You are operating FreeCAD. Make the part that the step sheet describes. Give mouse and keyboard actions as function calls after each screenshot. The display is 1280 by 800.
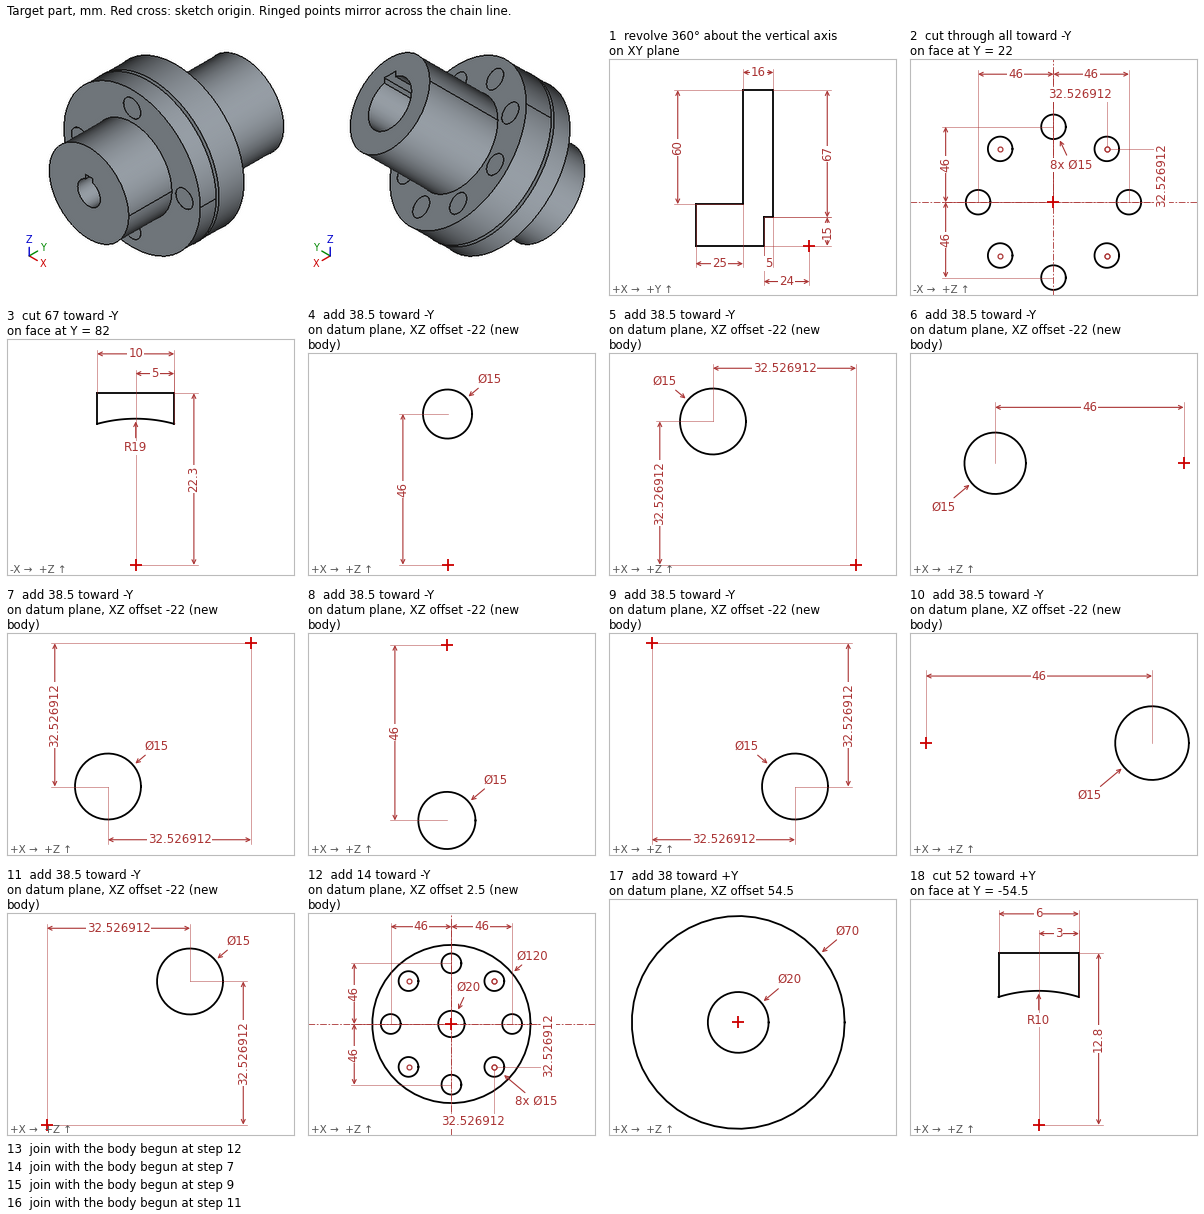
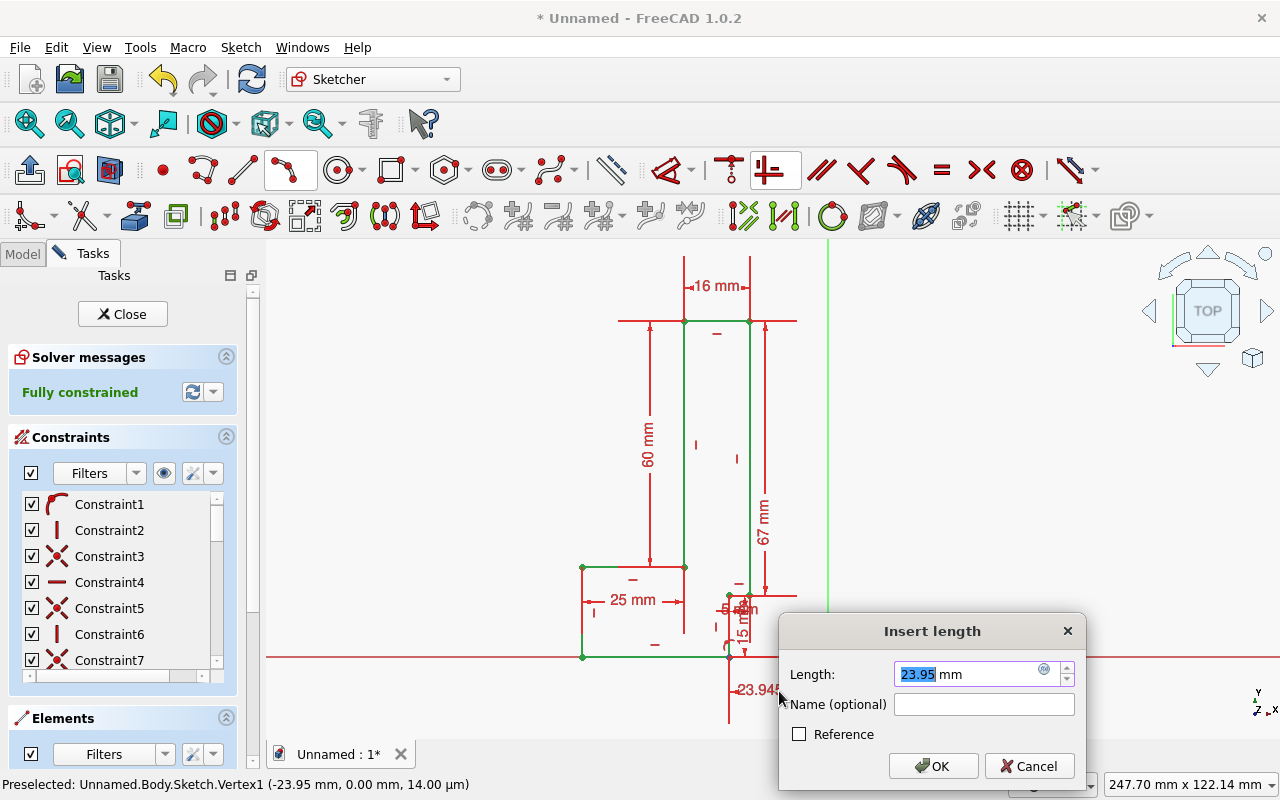
text(24)
key(Return)
key(Escape)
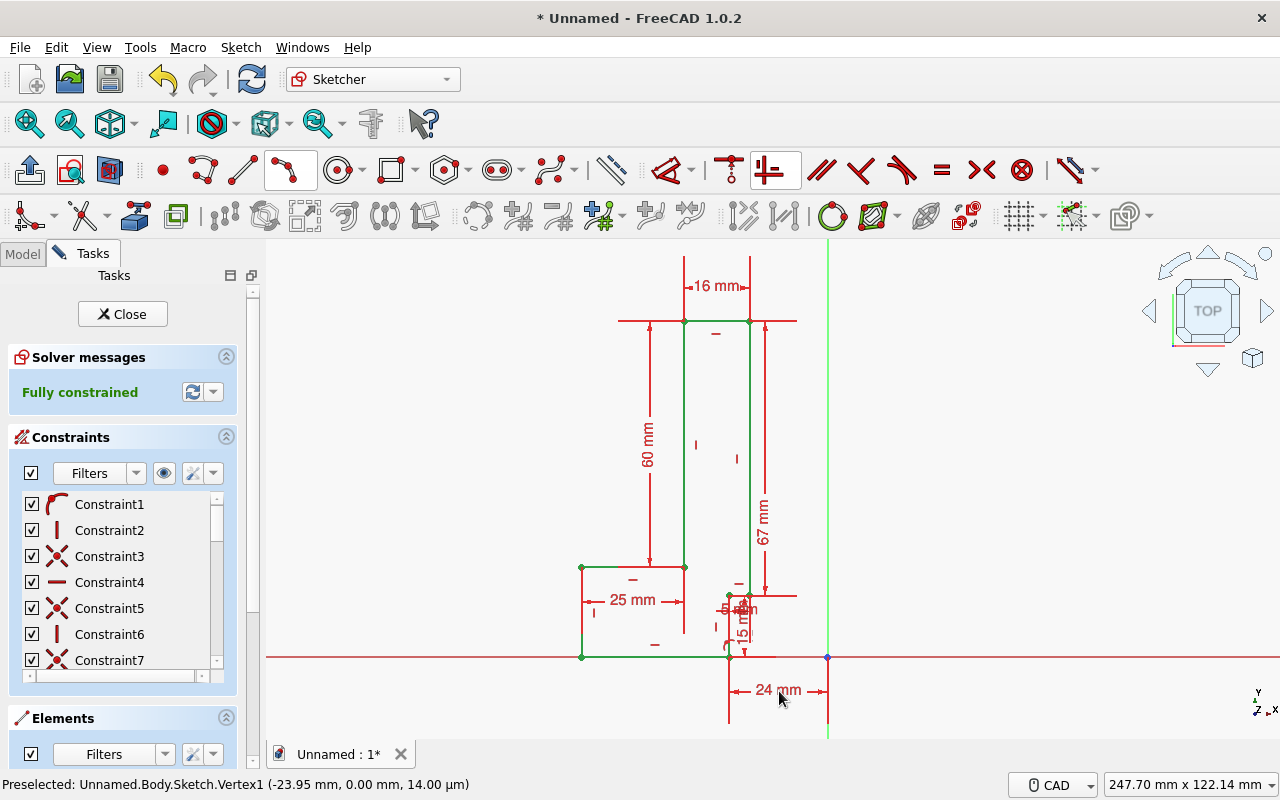
click(123, 314)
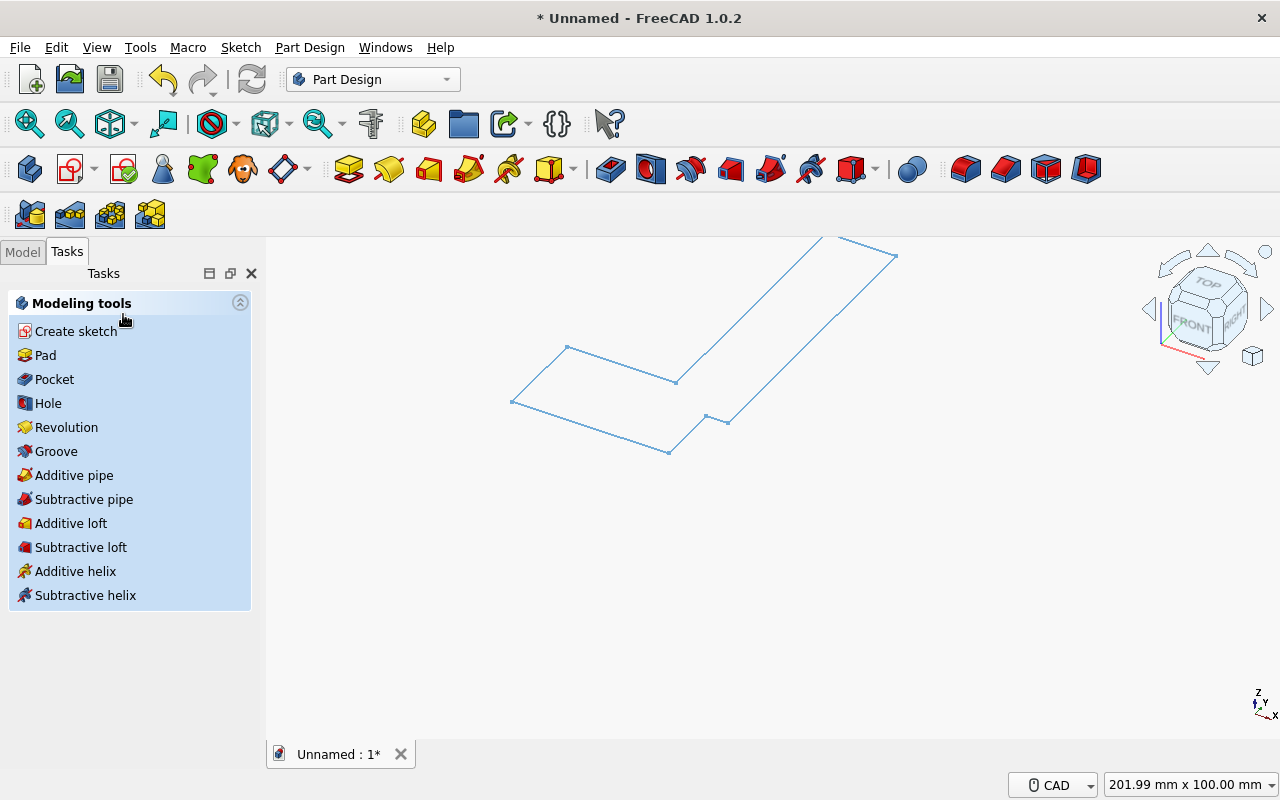
click(390, 170)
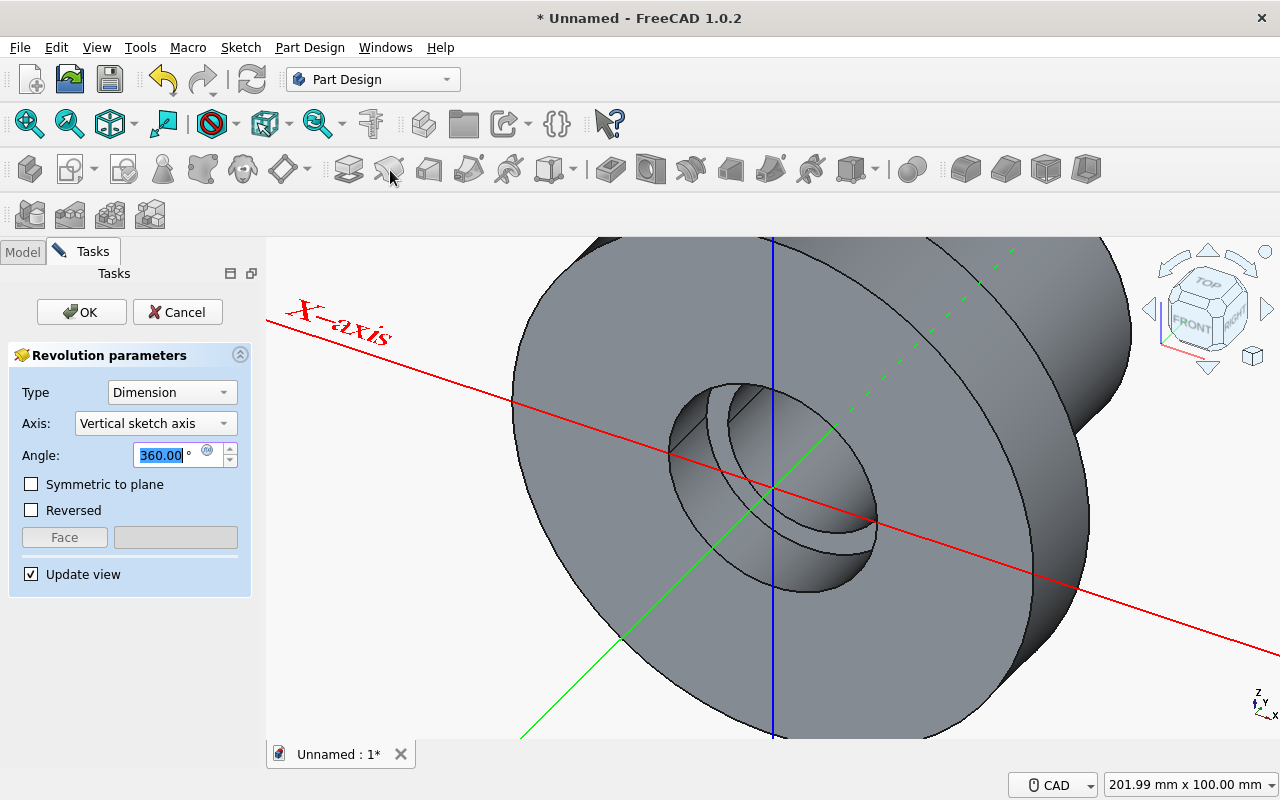
click(82, 312)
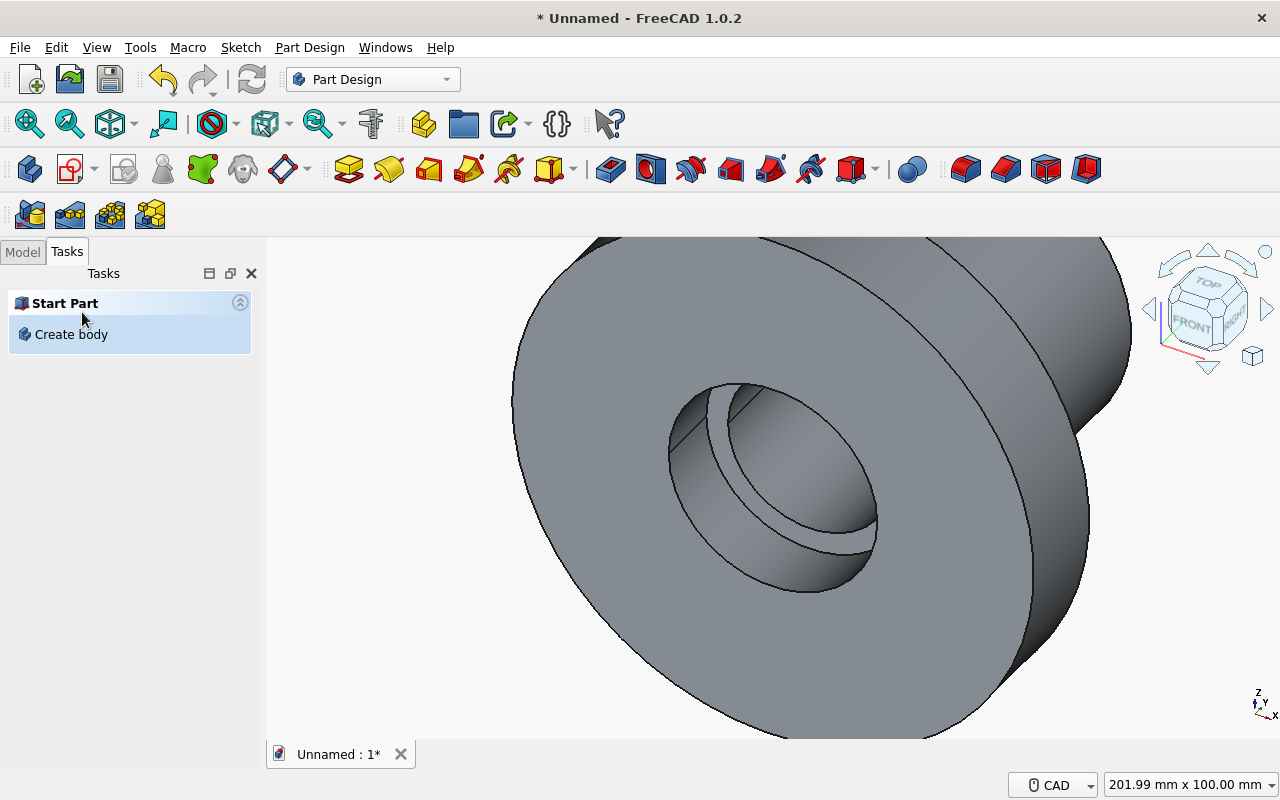
click(30, 124)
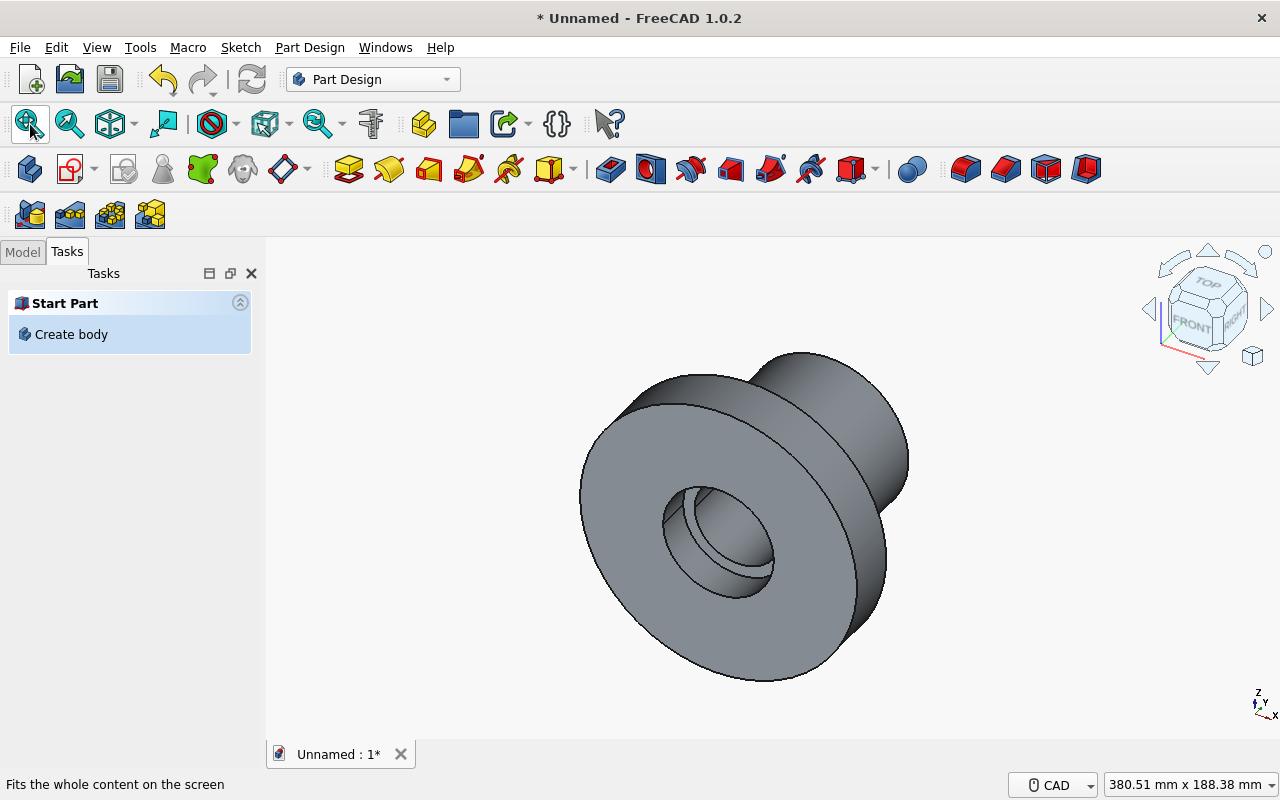
key(4)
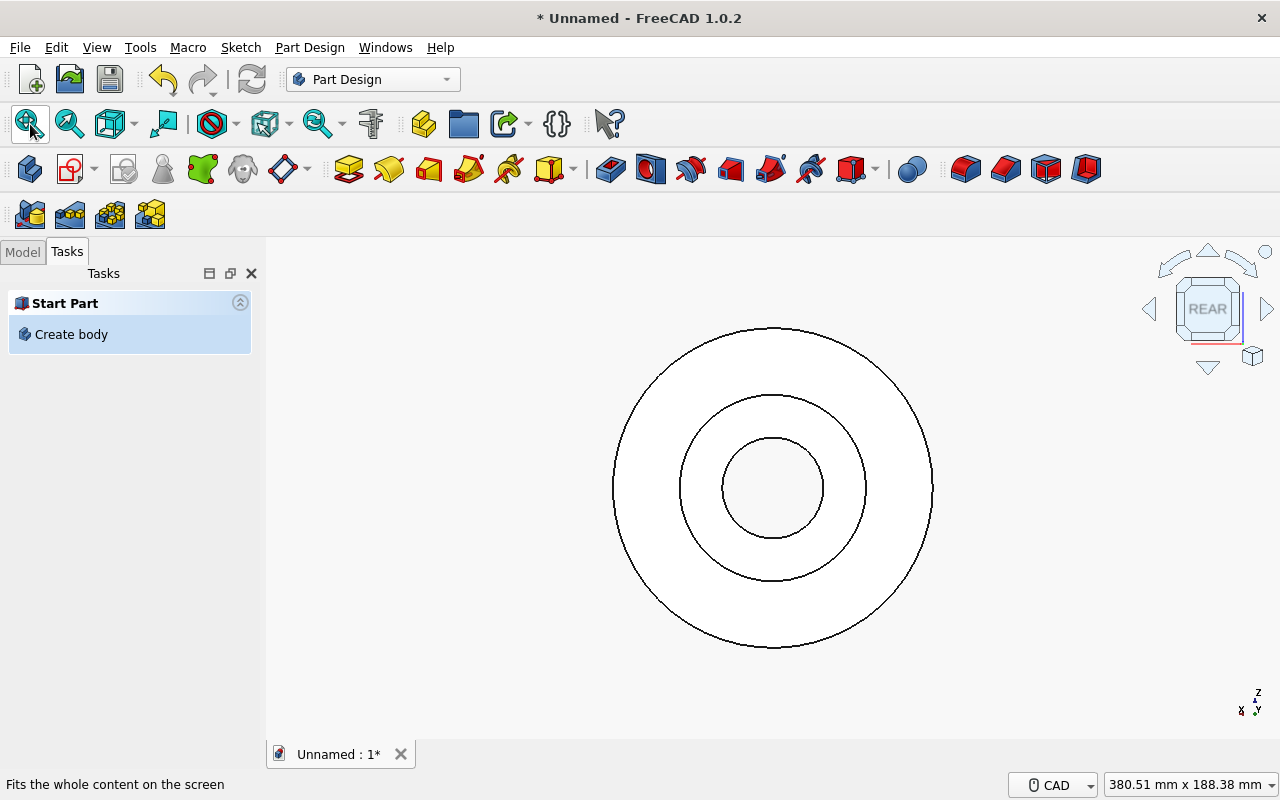
click(864, 578)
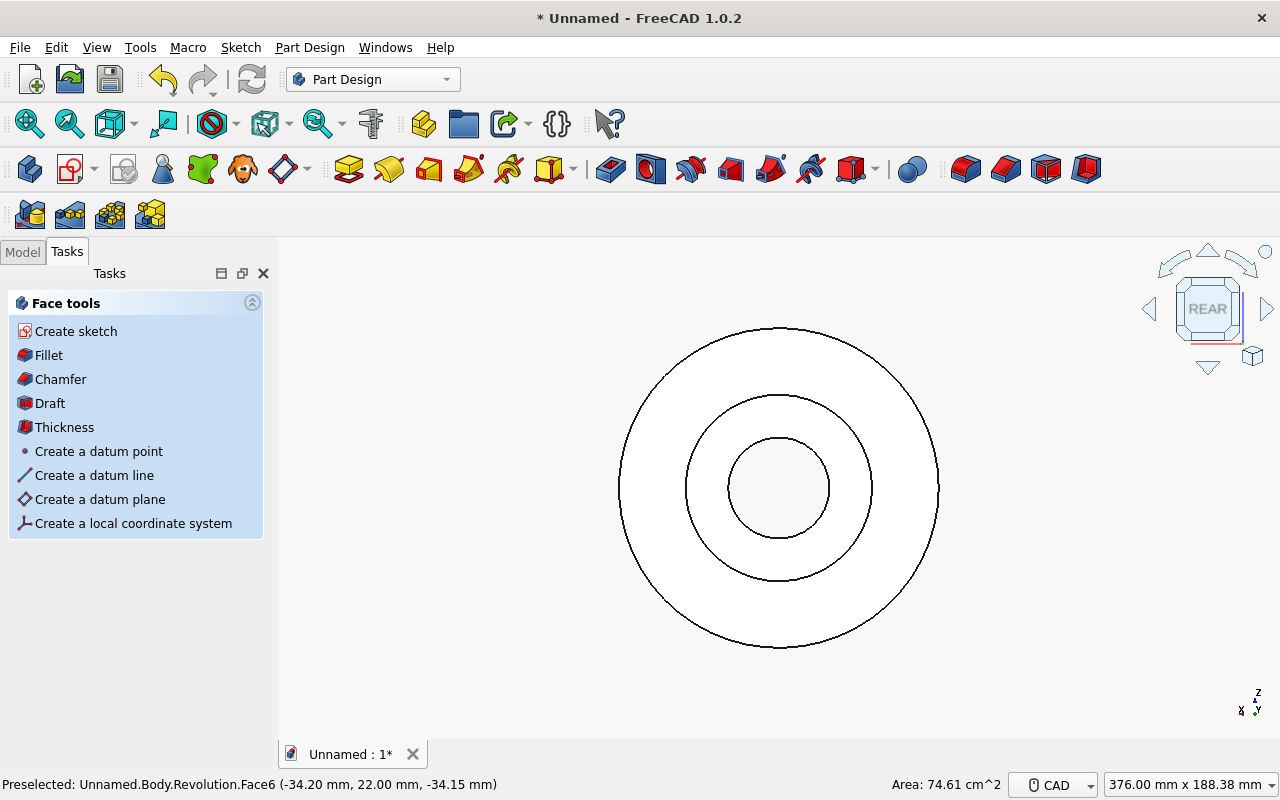
click(70, 170)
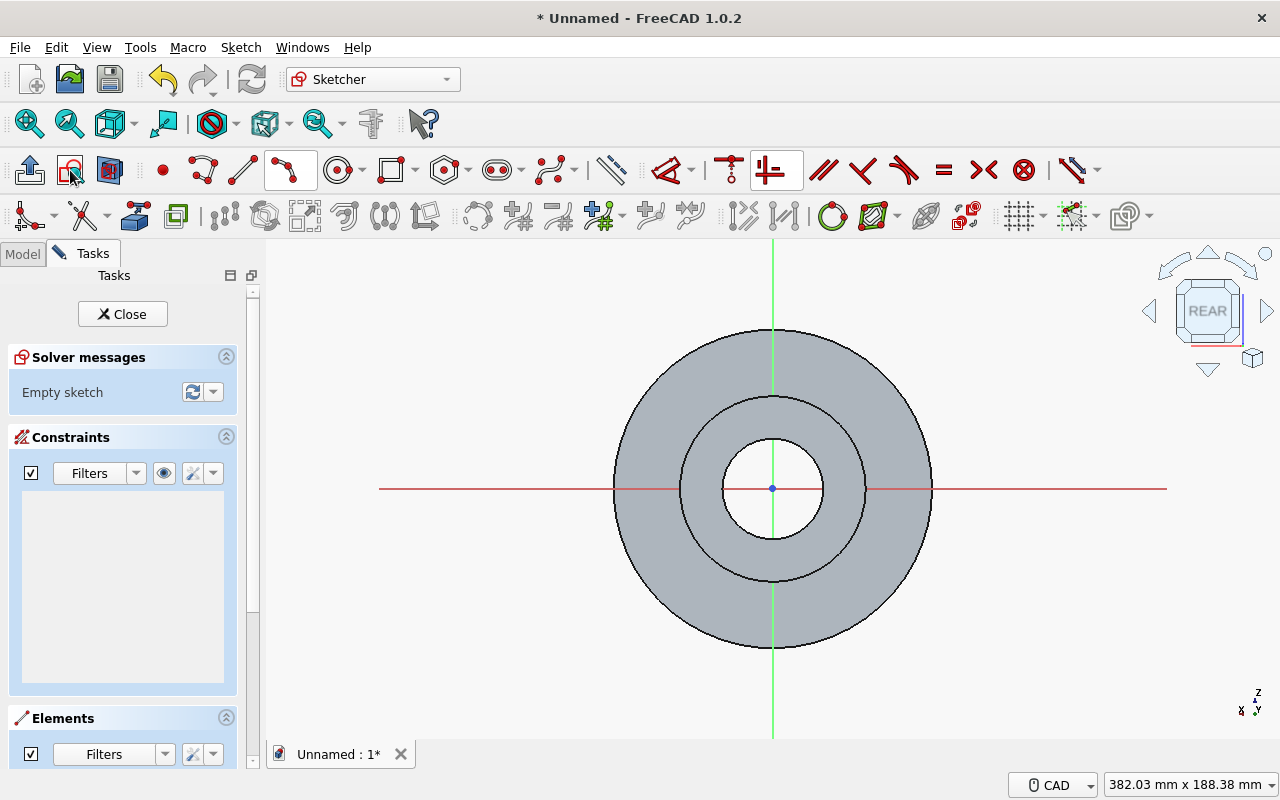
click(110, 170)